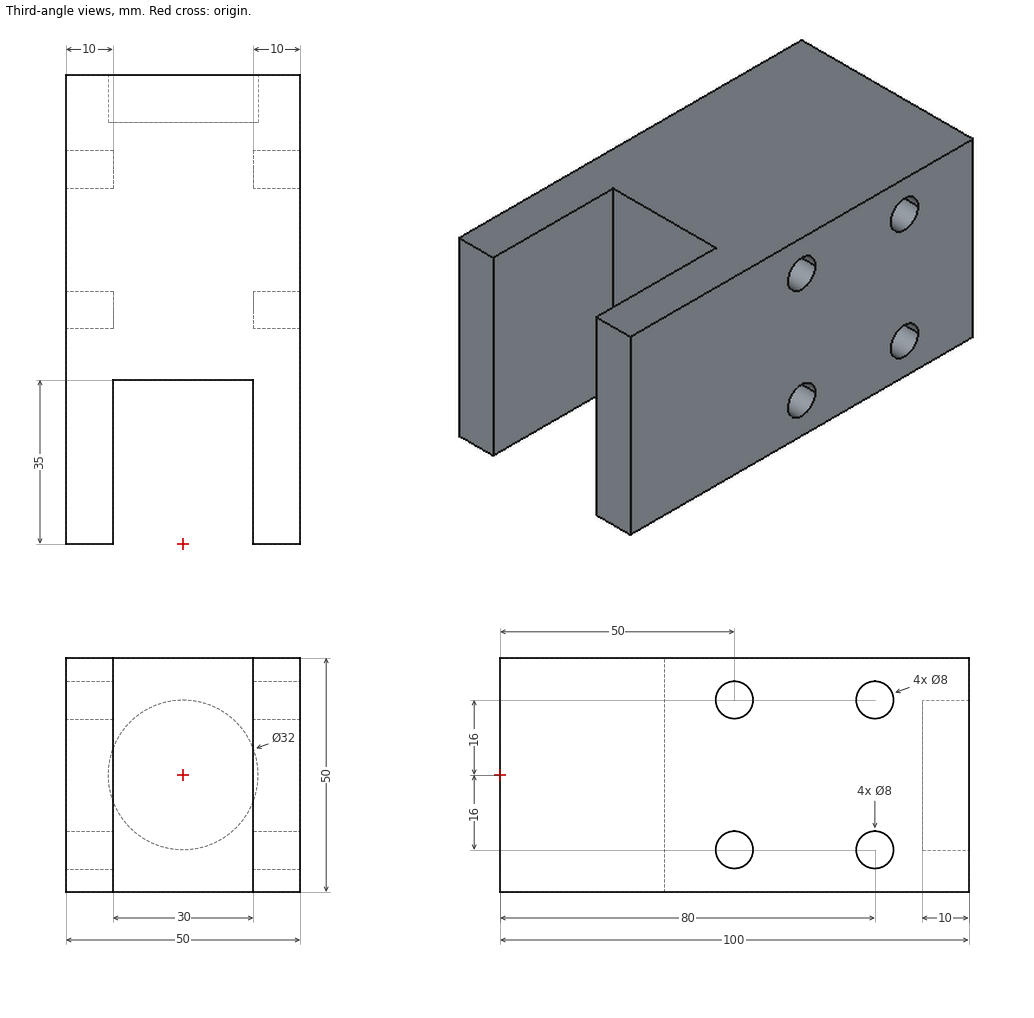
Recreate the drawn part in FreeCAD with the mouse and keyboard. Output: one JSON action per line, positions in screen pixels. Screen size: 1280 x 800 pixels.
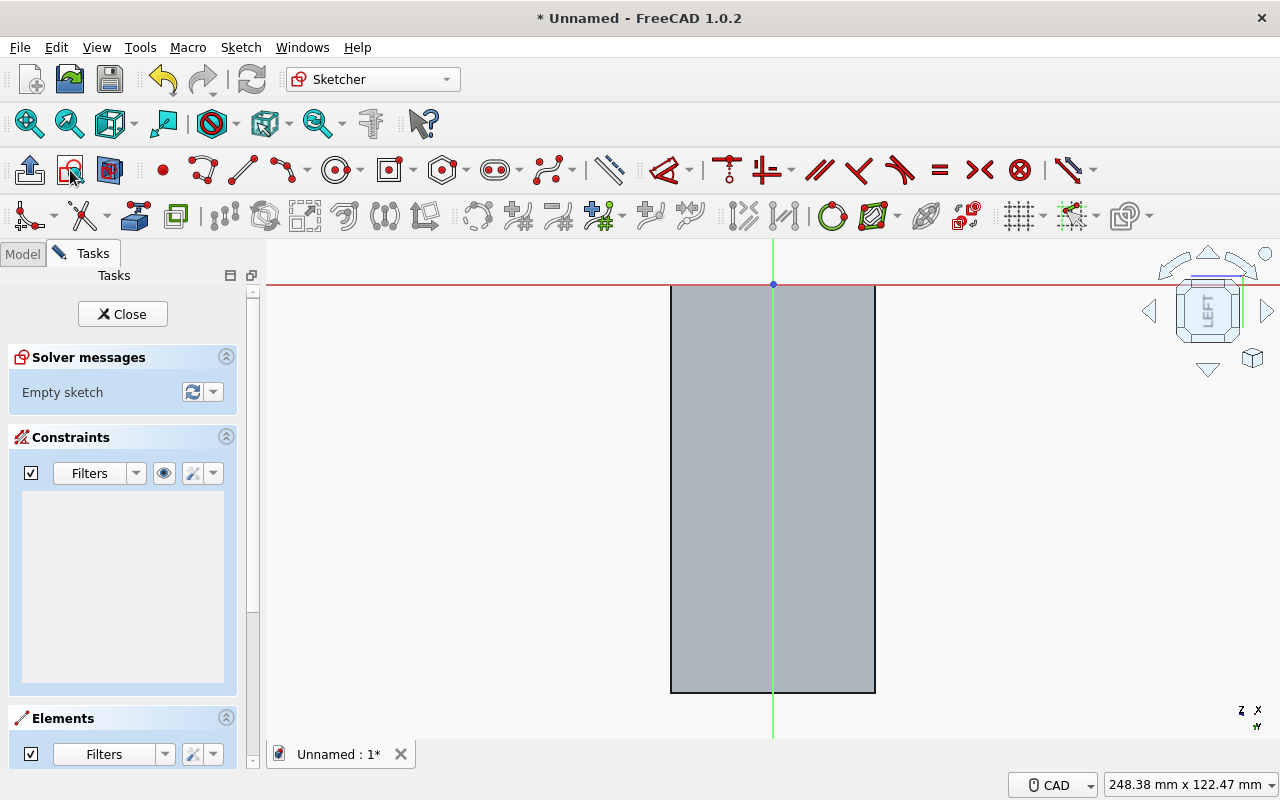
{"action": "scroll", "coordinate": [395, 637], "scroll_direction": "down", "scroll_amount": 1}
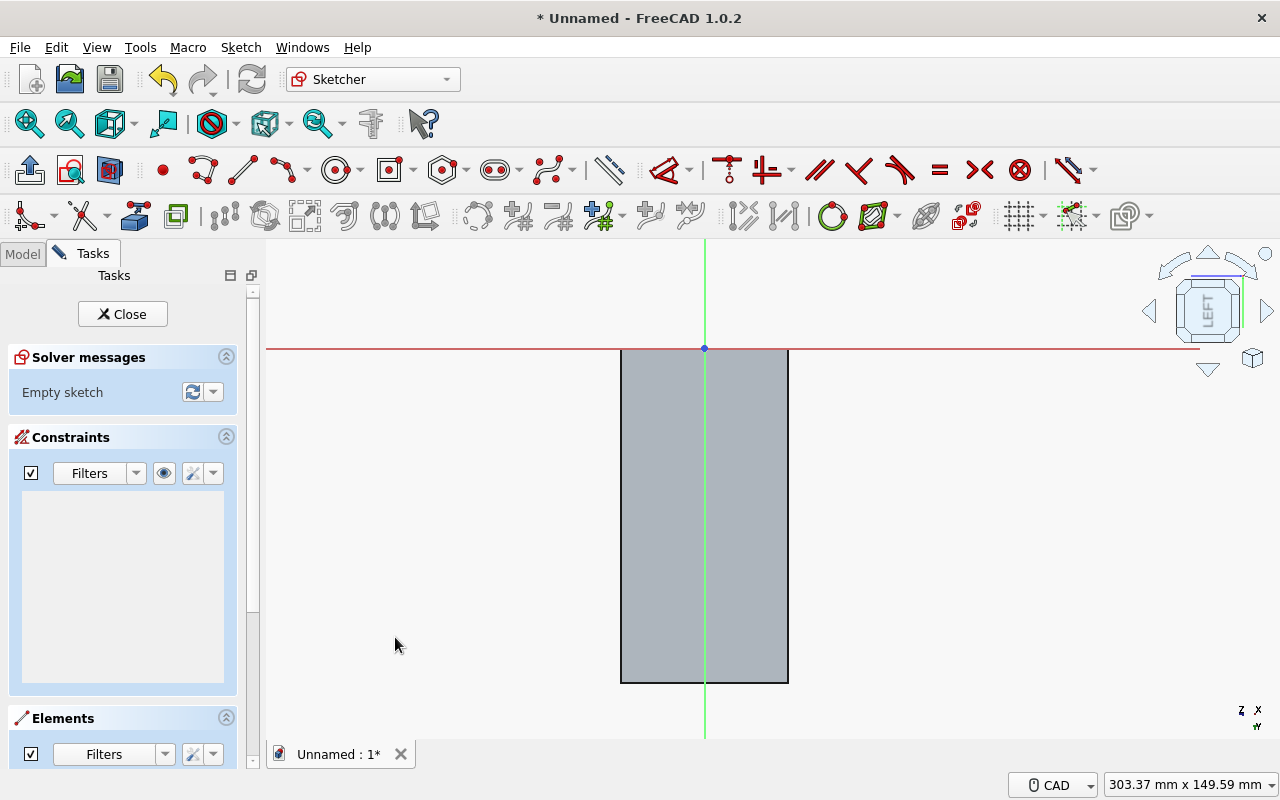
{"action": "left_click", "coordinate": [336, 170]}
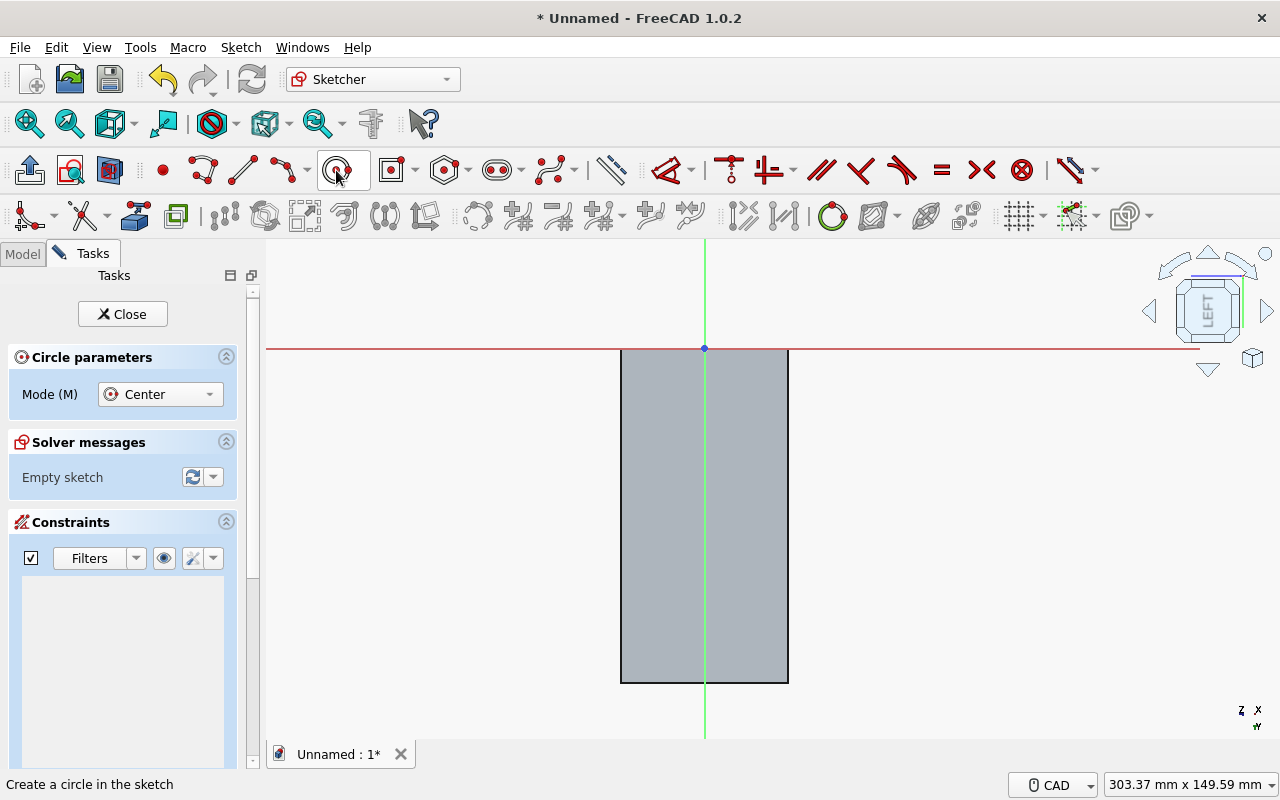
{"action": "scroll", "coordinate": [758, 616], "scroll_direction": "up", "scroll_amount": 3}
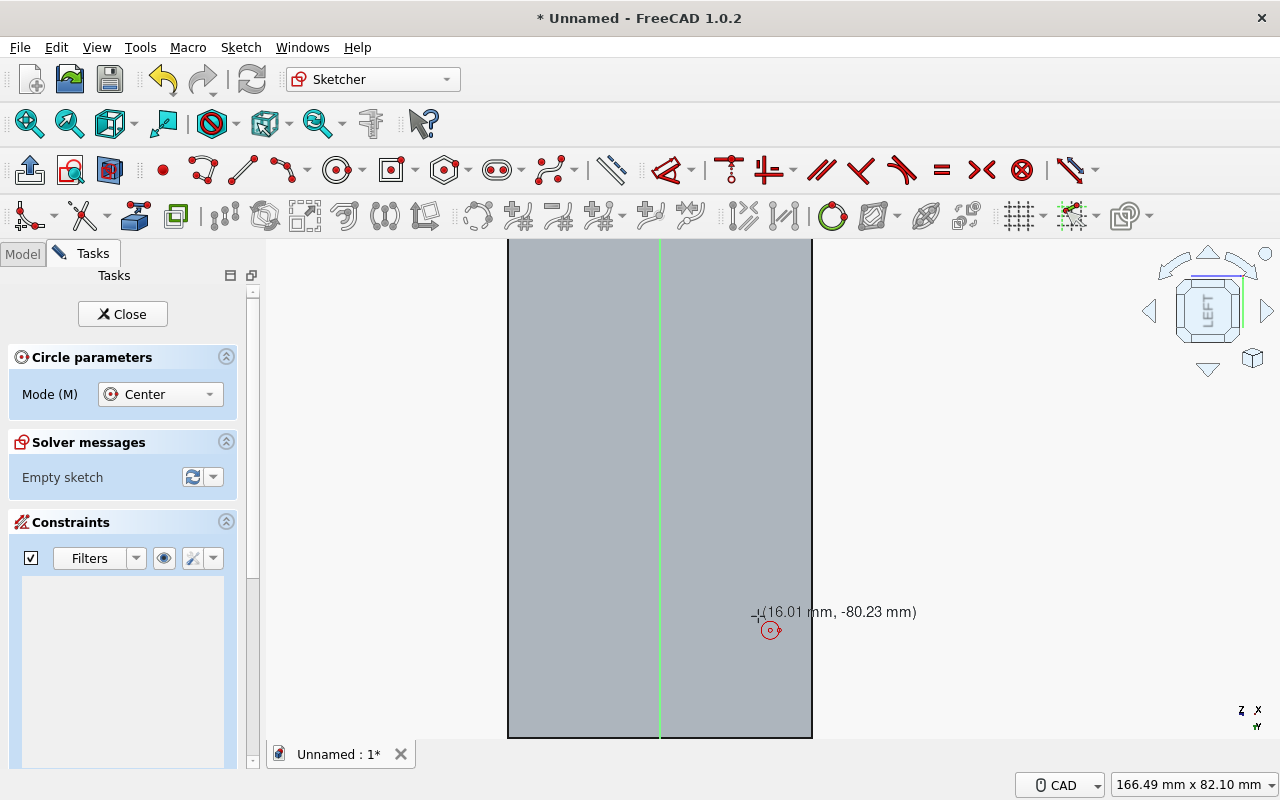
{"action": "left_click", "coordinate": [758, 616]}
{"action": "mouse_move", "coordinate": [775, 599]}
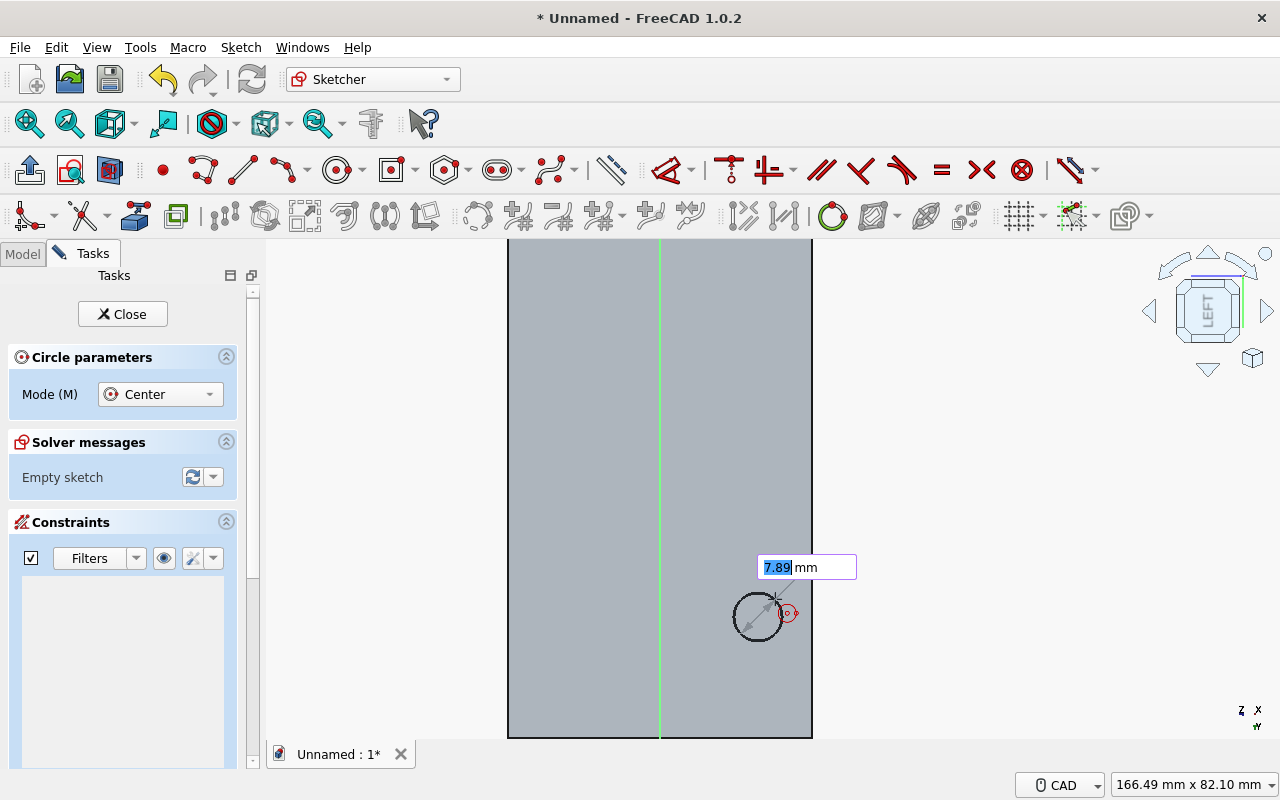
{"action": "type", "text": "8"}
{"action": "key", "text": "Return"}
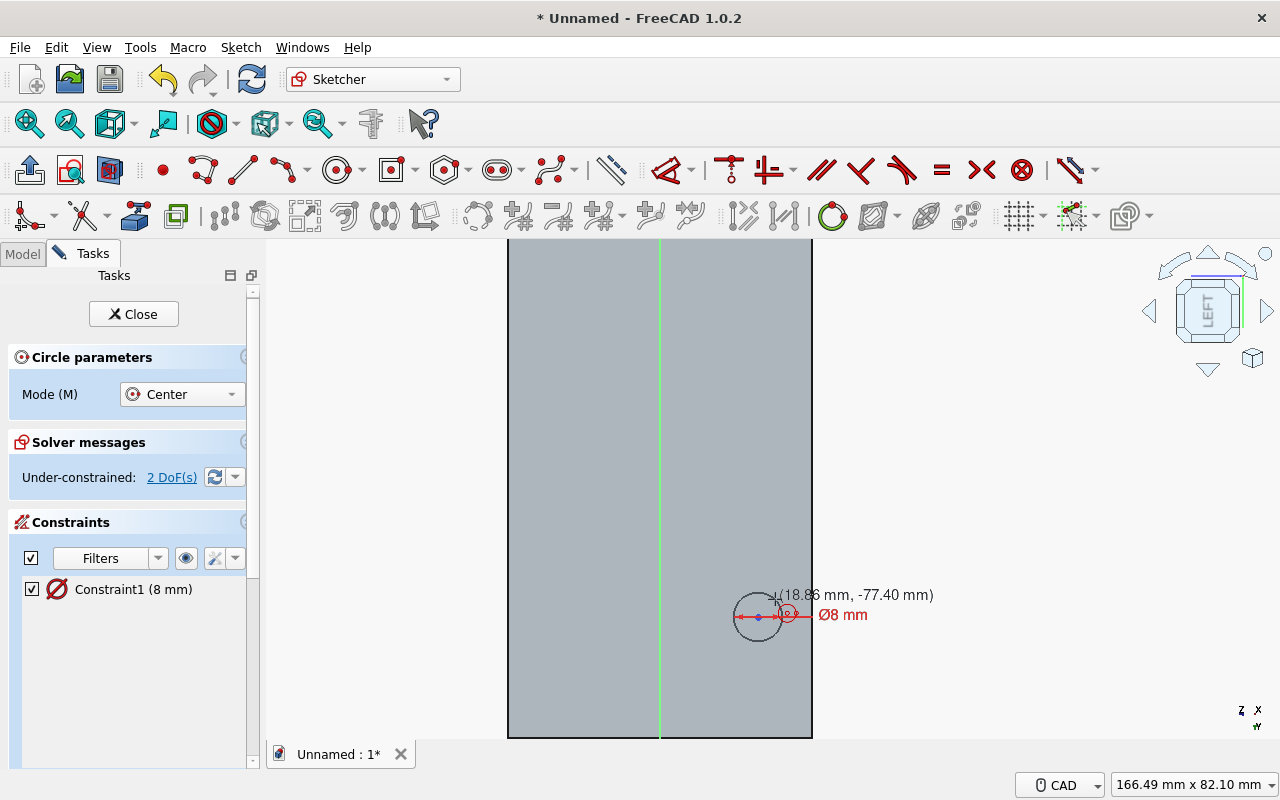
{"action": "left_click", "coordinate": [563, 616]}
{"action": "mouse_move", "coordinate": [580, 599]}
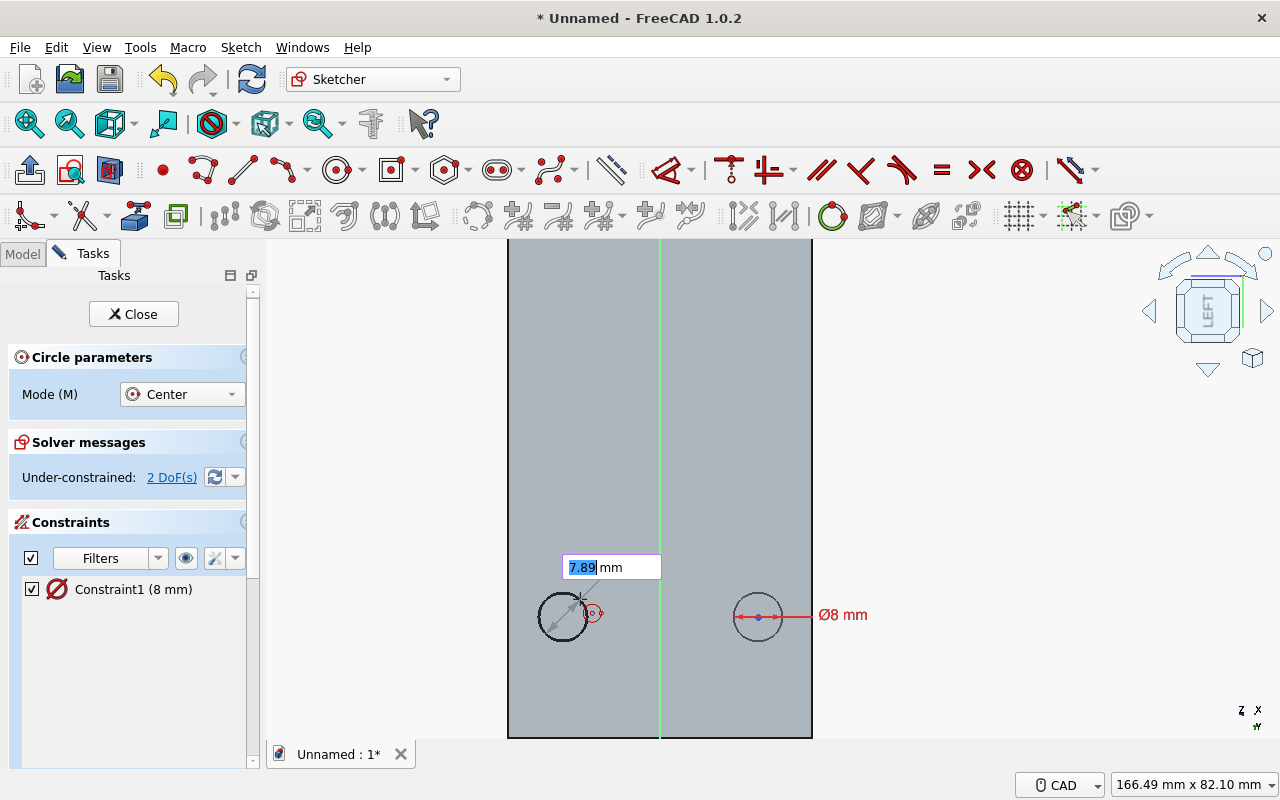
{"action": "type", "text": "8"}
{"action": "key", "text": "Return"}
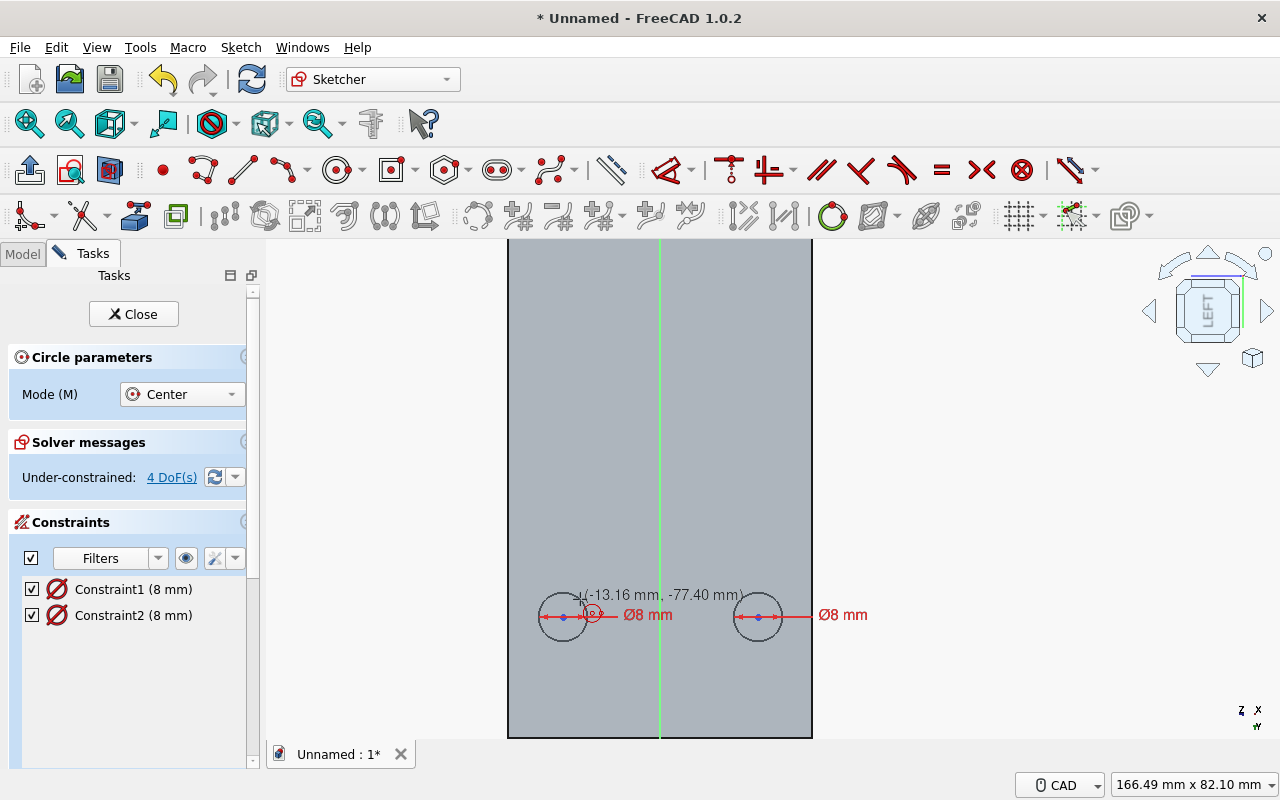
{"action": "left_click", "coordinate": [563, 433]}
{"action": "mouse_move", "coordinate": [580, 416]}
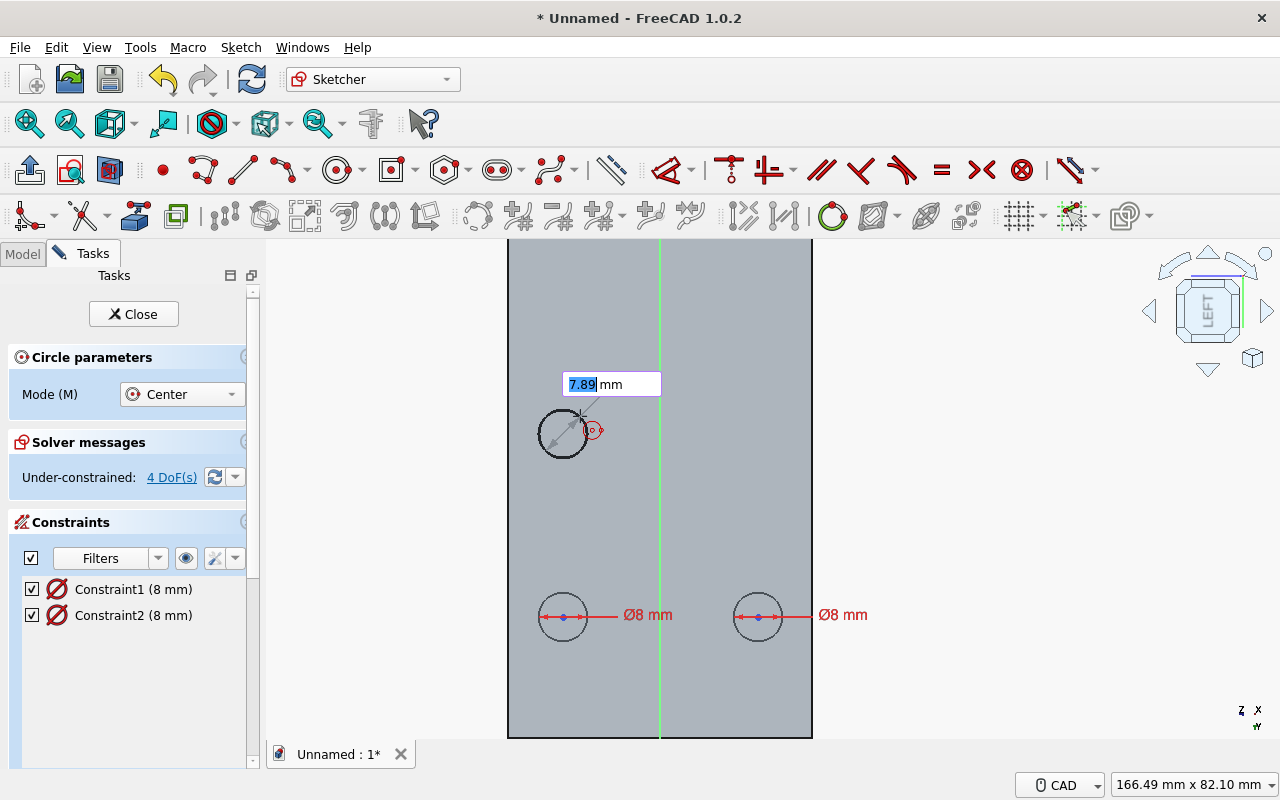
{"action": "type", "text": "8"}
{"action": "key", "text": "Return"}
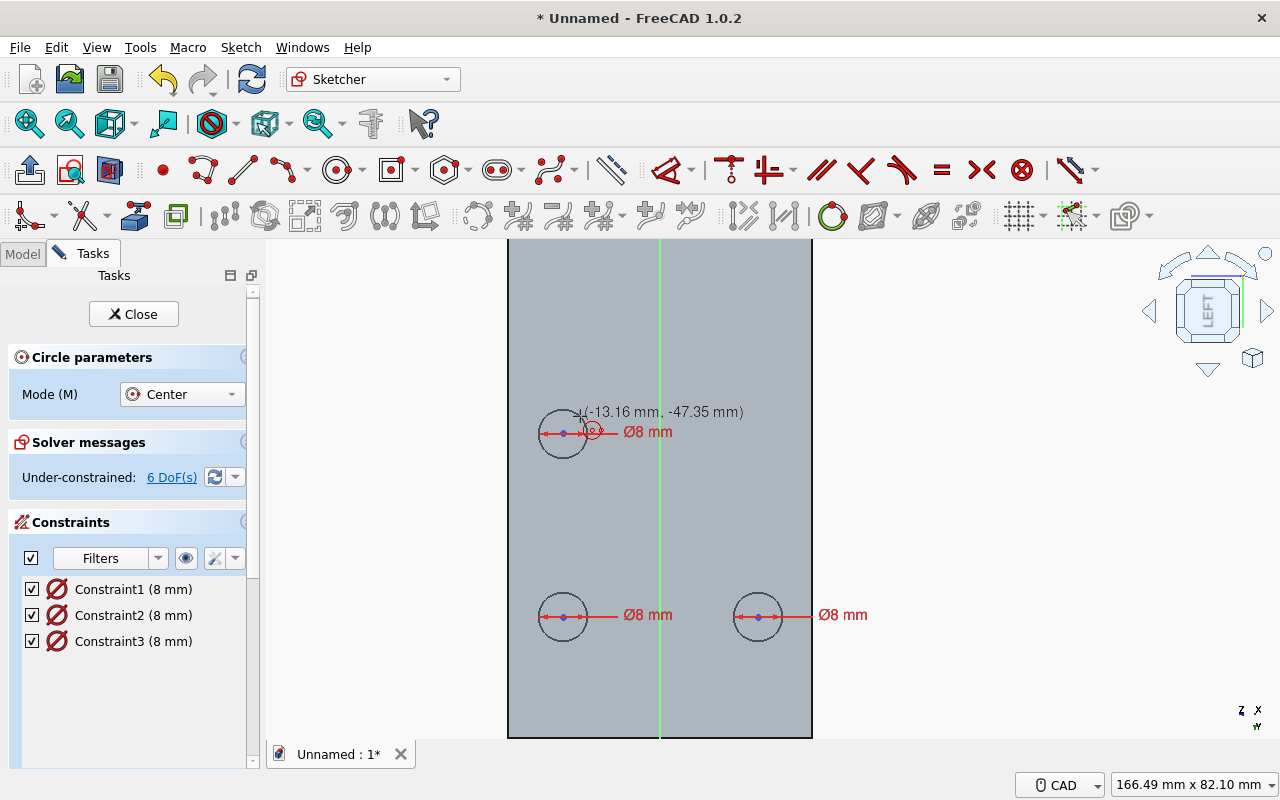
{"action": "left_click", "coordinate": [758, 433]}
{"action": "mouse_move", "coordinate": [775, 416]}